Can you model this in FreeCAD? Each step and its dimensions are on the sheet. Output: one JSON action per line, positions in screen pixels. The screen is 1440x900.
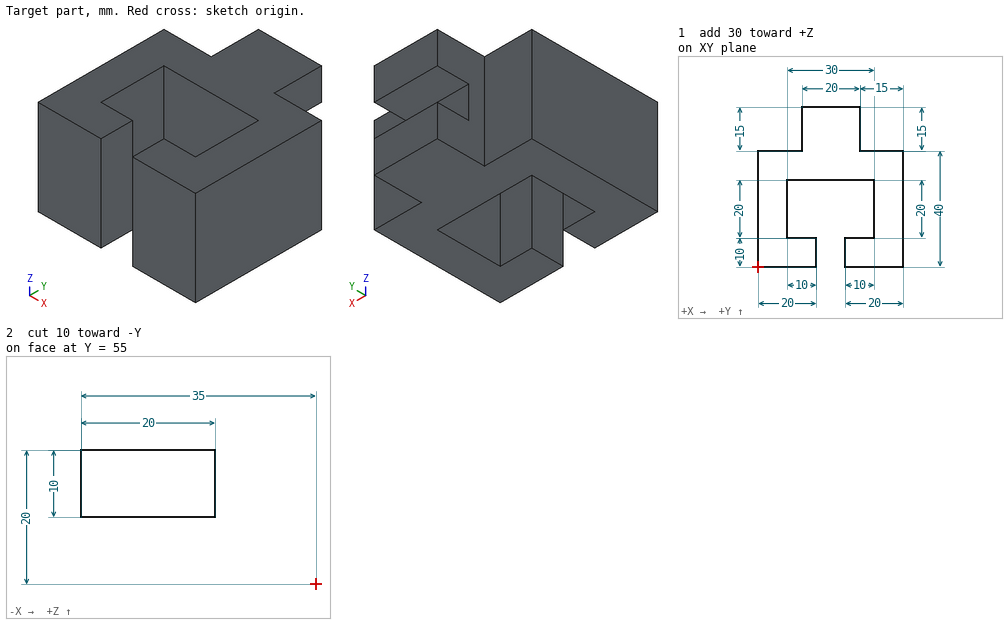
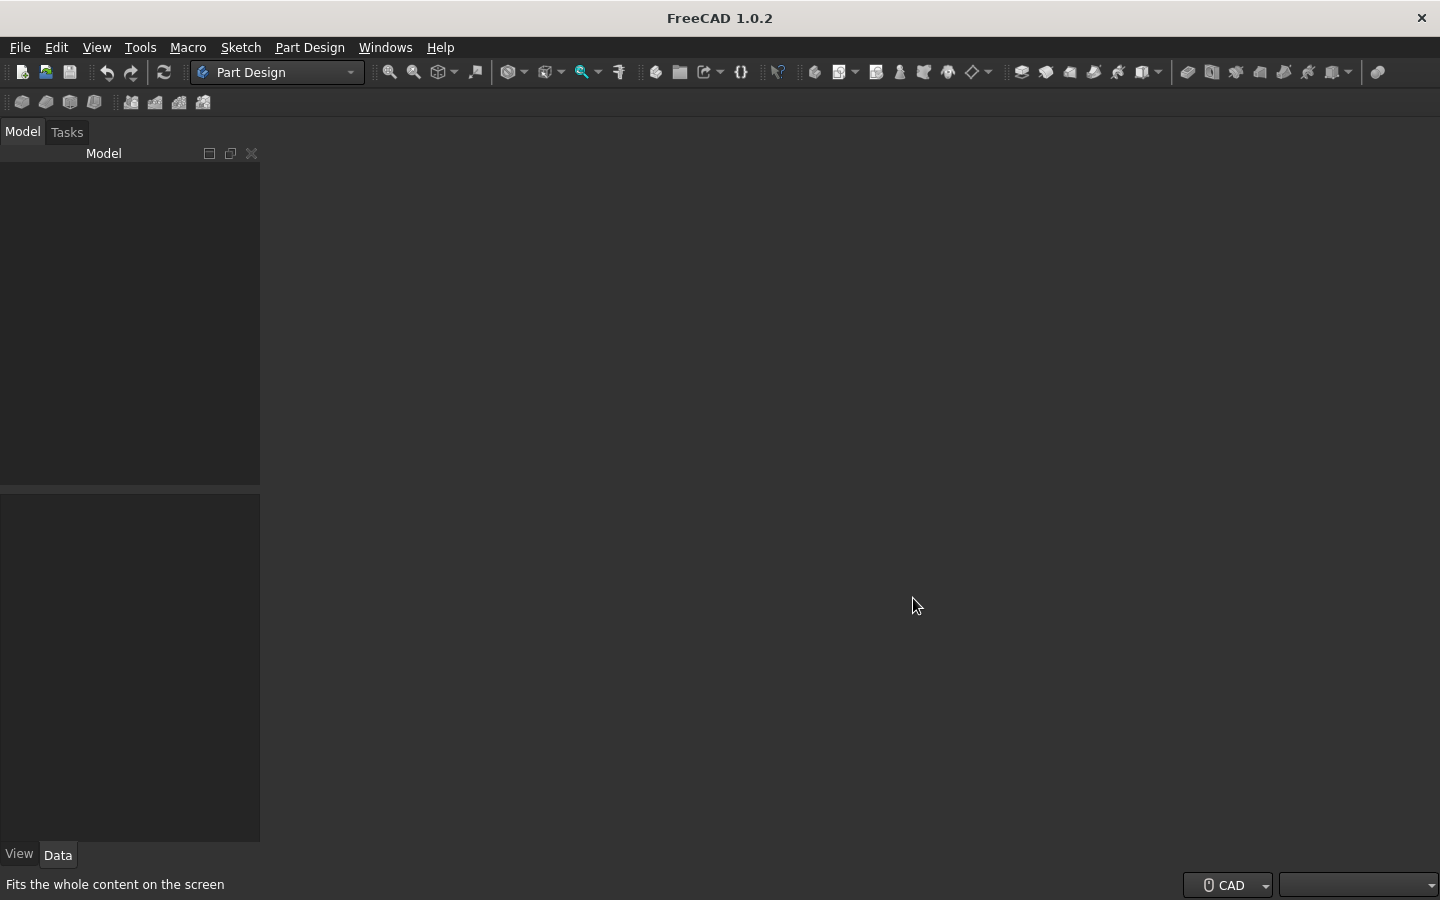
{"action": "left_click", "coordinate": [22, 72]}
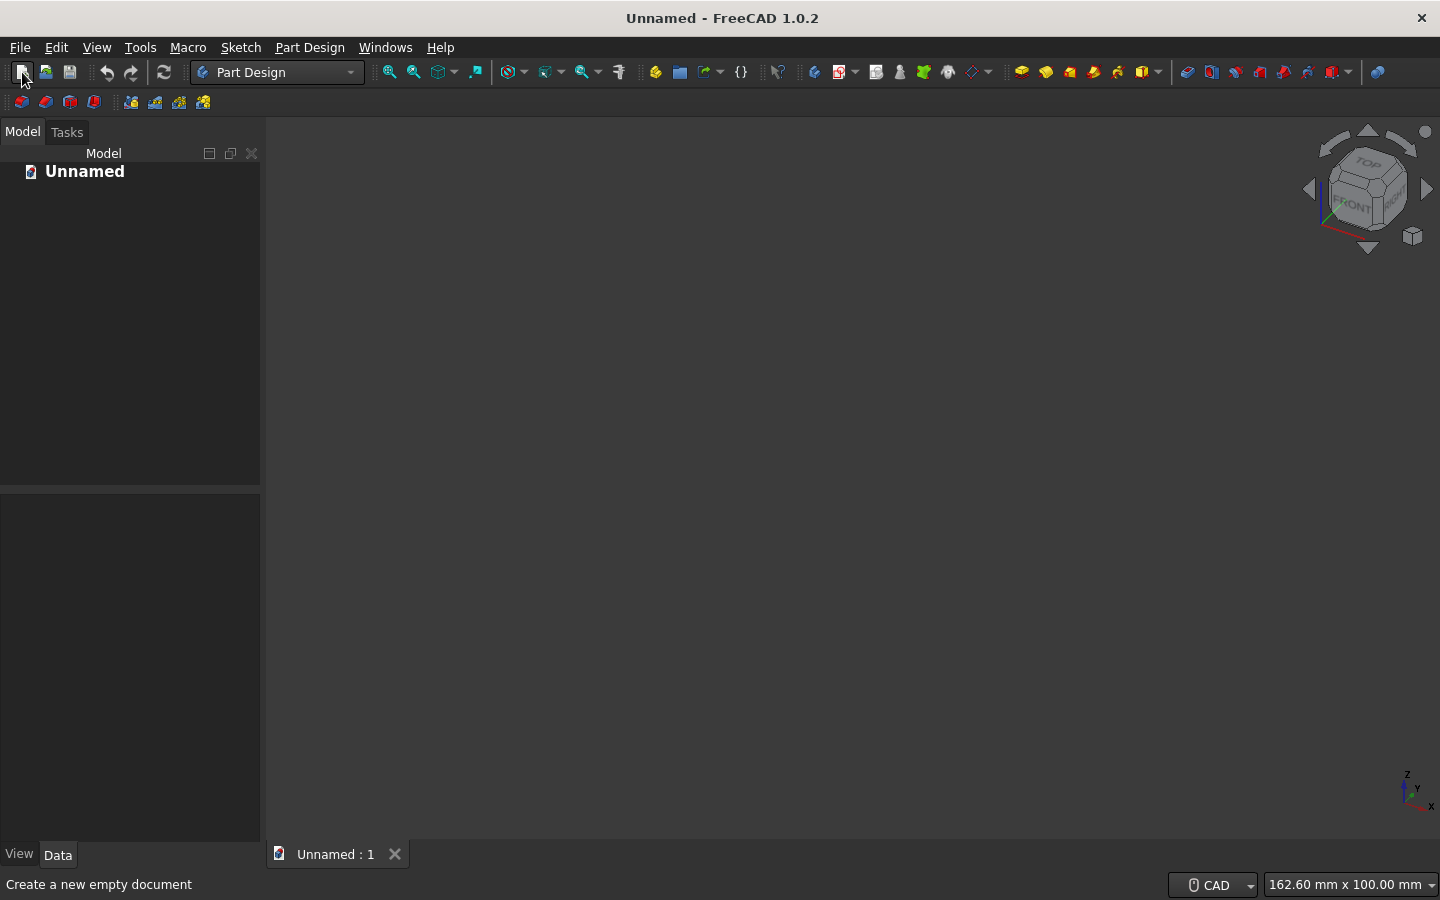
{"action": "left_click", "coordinate": [840, 72]}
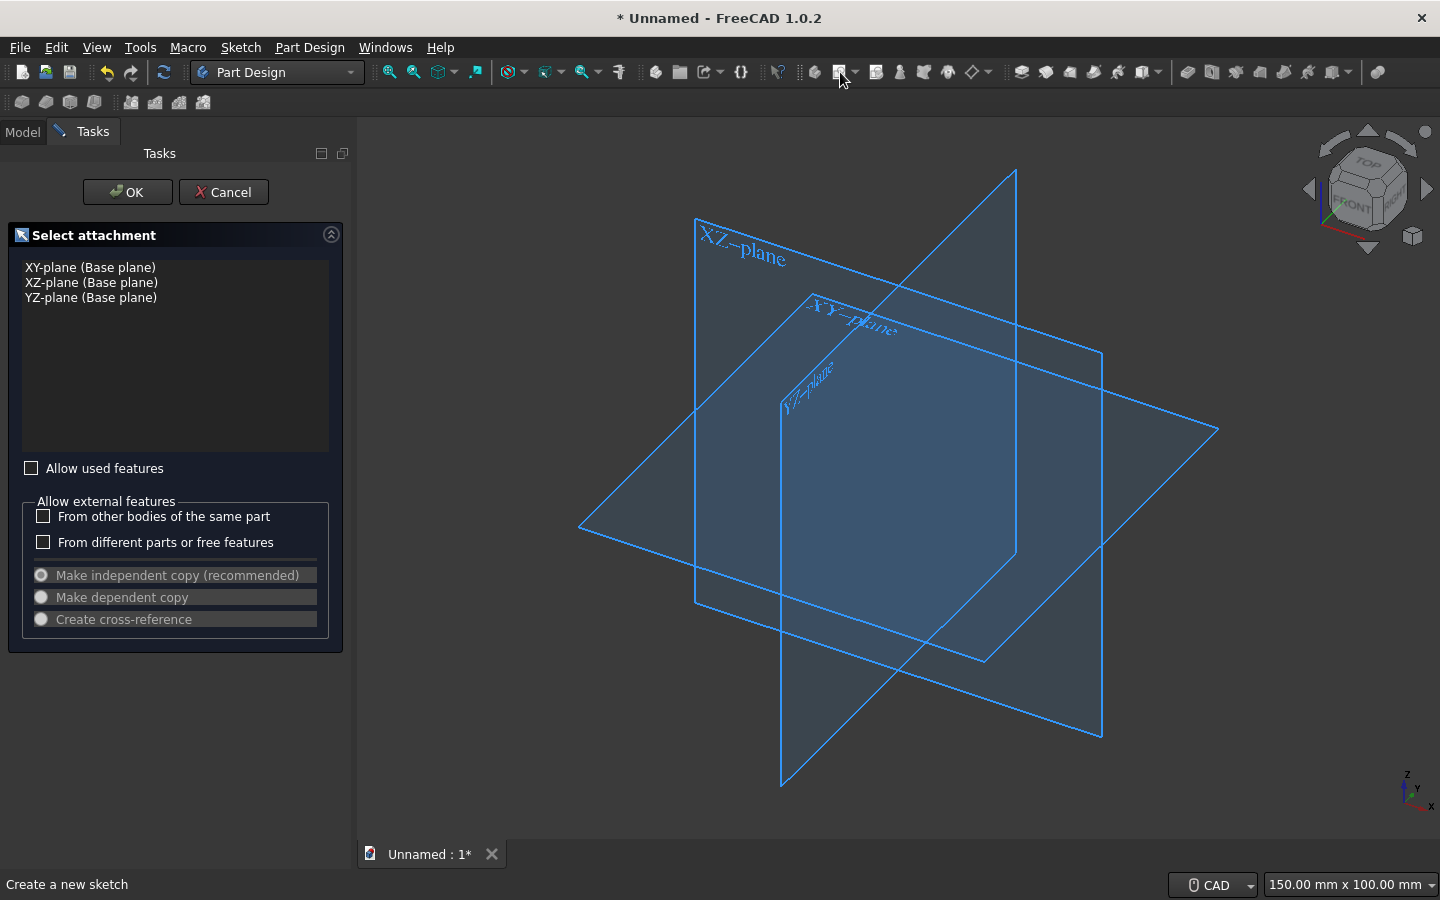
{"action": "left_click", "coordinate": [82, 268]}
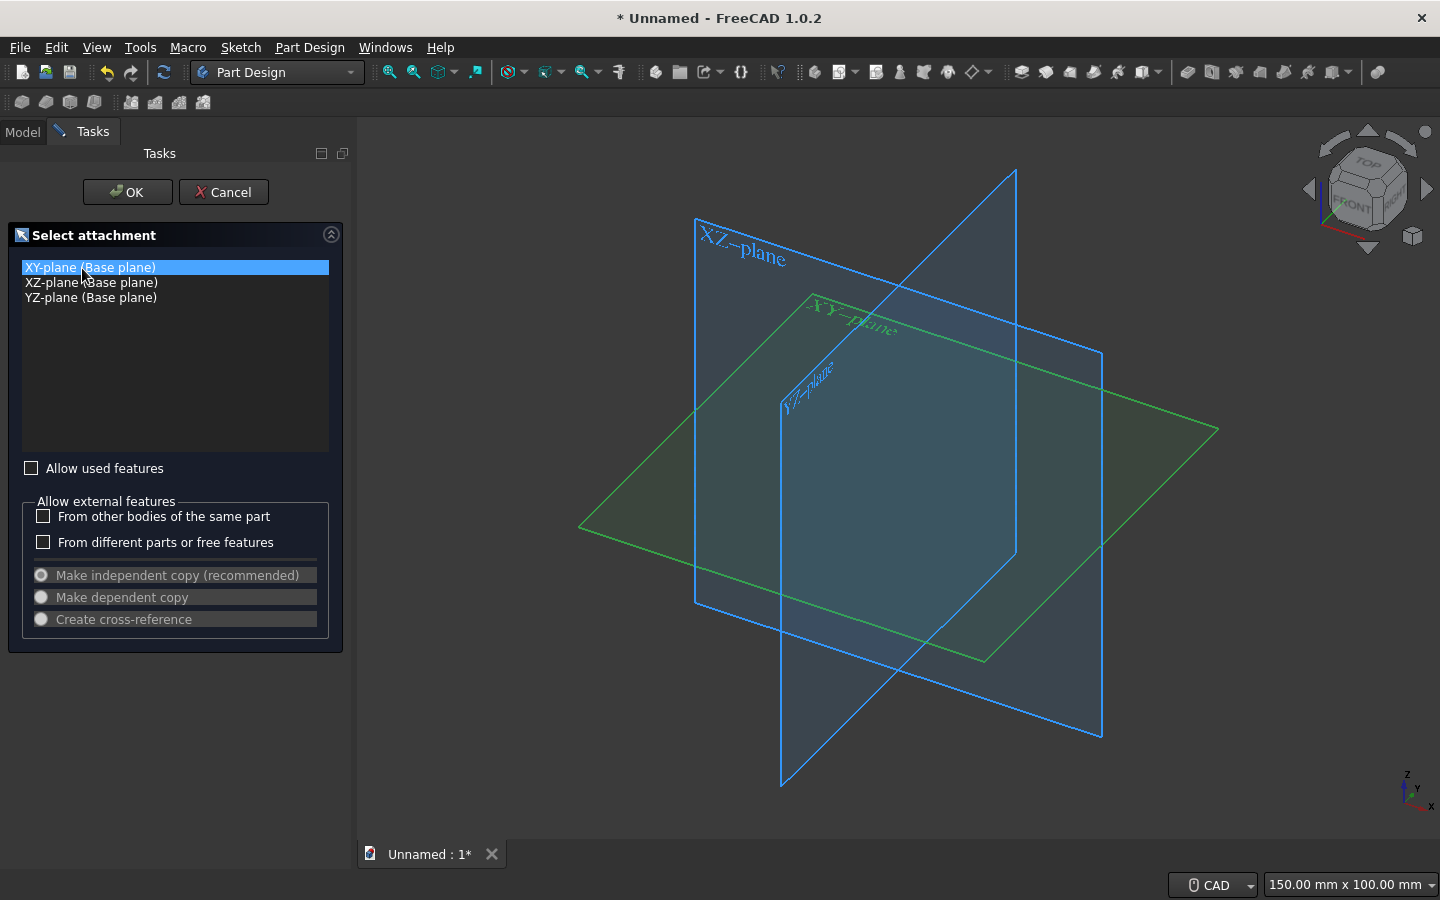
{"action": "left_click", "coordinate": [128, 192]}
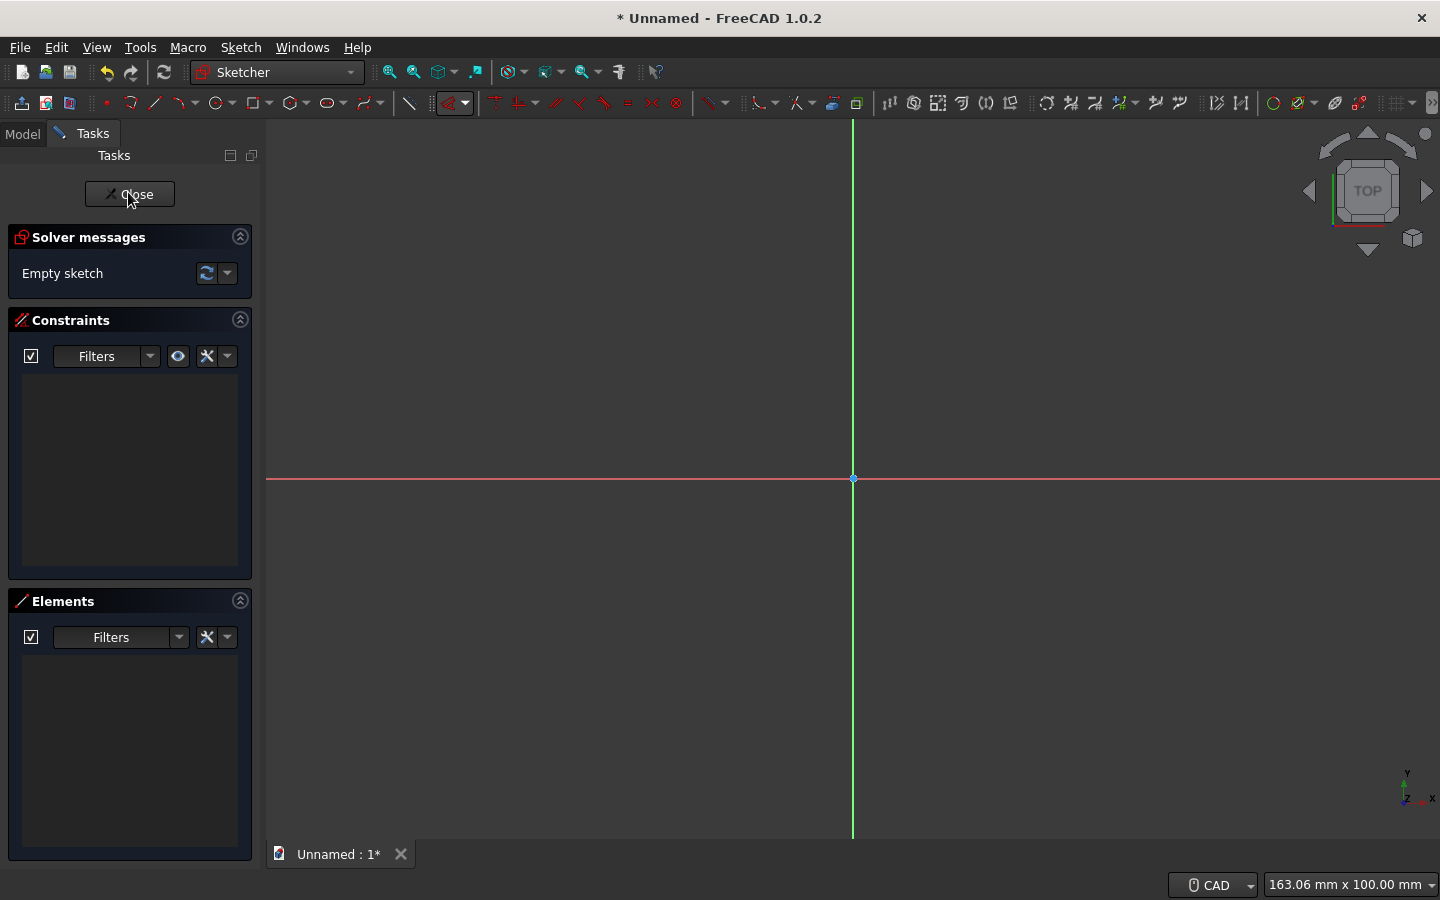
{"action": "scroll", "coordinate": [294, 811], "scroll_direction": "down", "scroll_amount": 1}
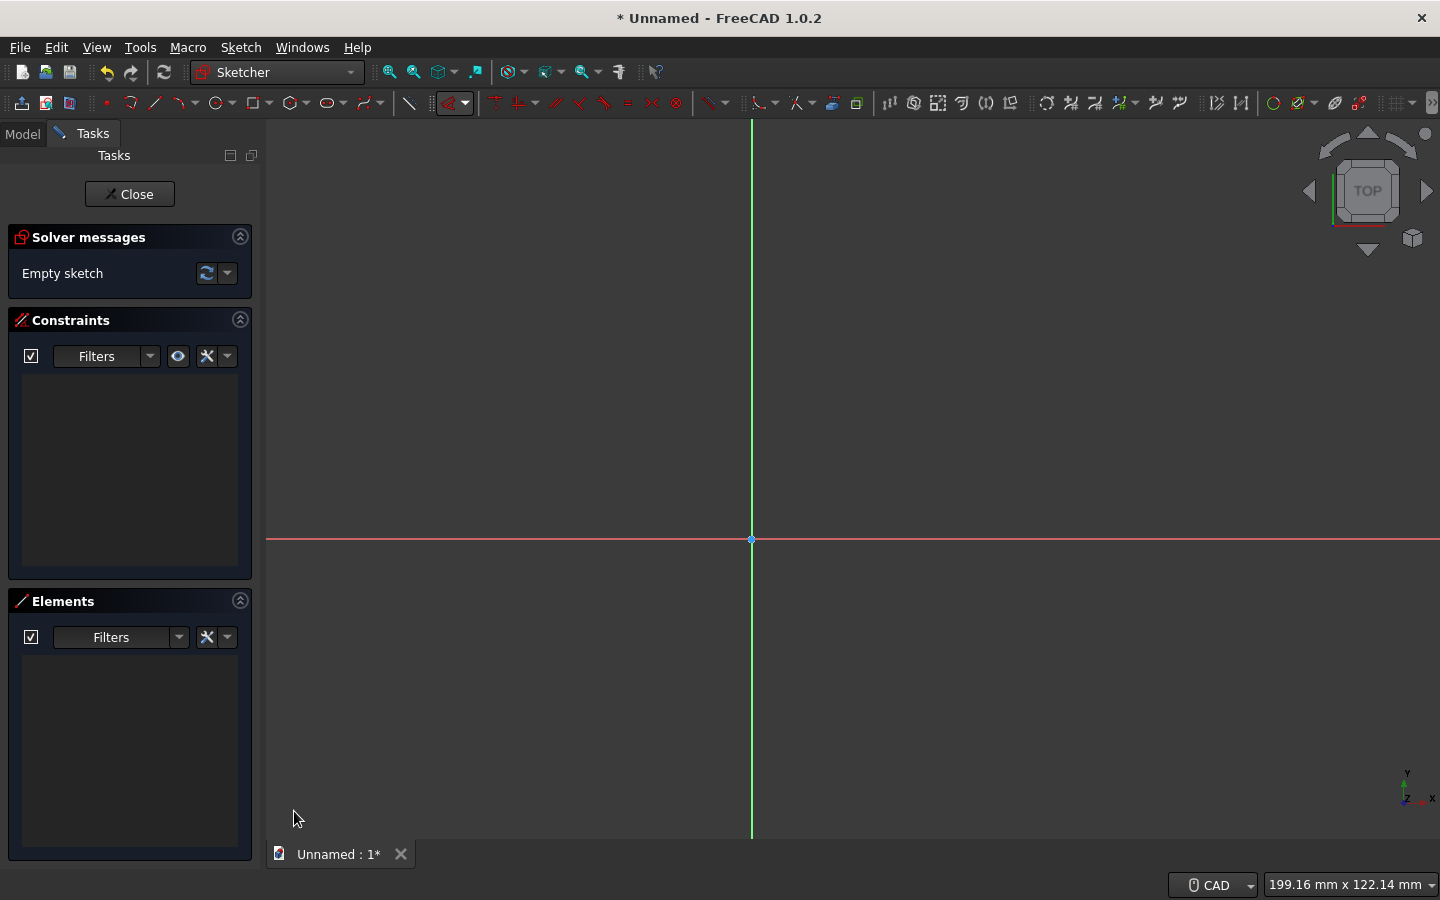
{"action": "scroll", "coordinate": [1132, 170], "scroll_direction": "up", "scroll_amount": 2}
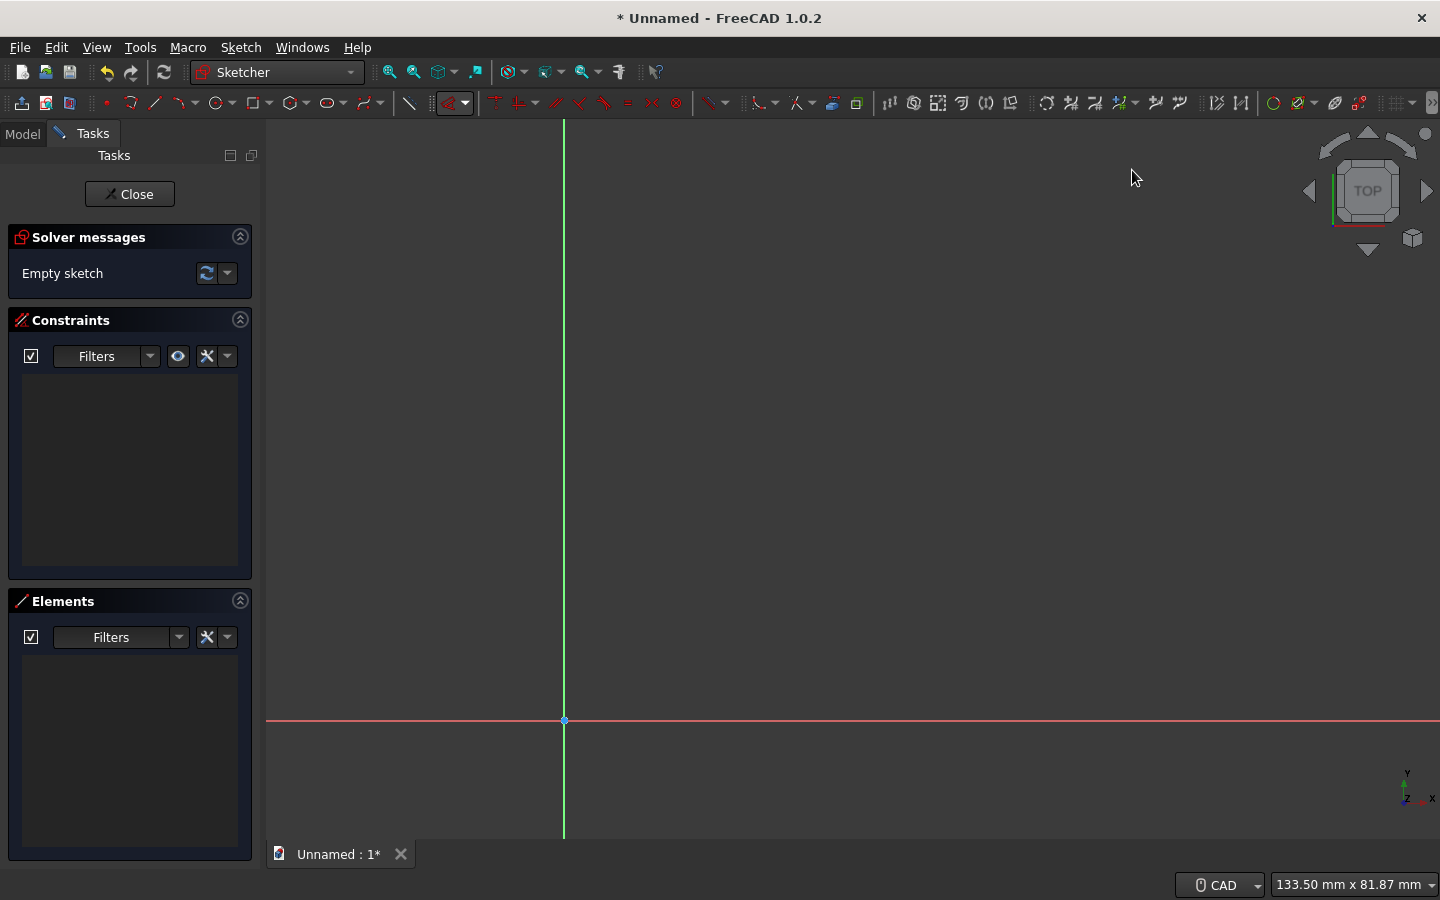
{"action": "left_click", "coordinate": [132, 104]}